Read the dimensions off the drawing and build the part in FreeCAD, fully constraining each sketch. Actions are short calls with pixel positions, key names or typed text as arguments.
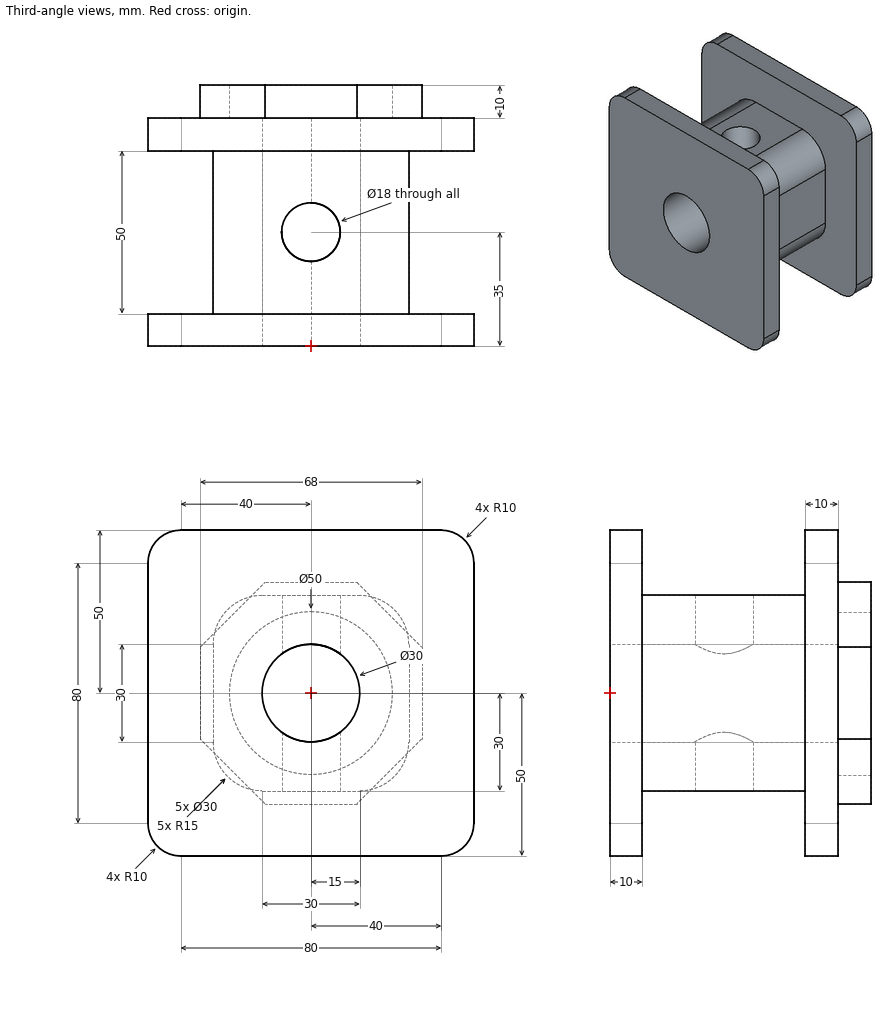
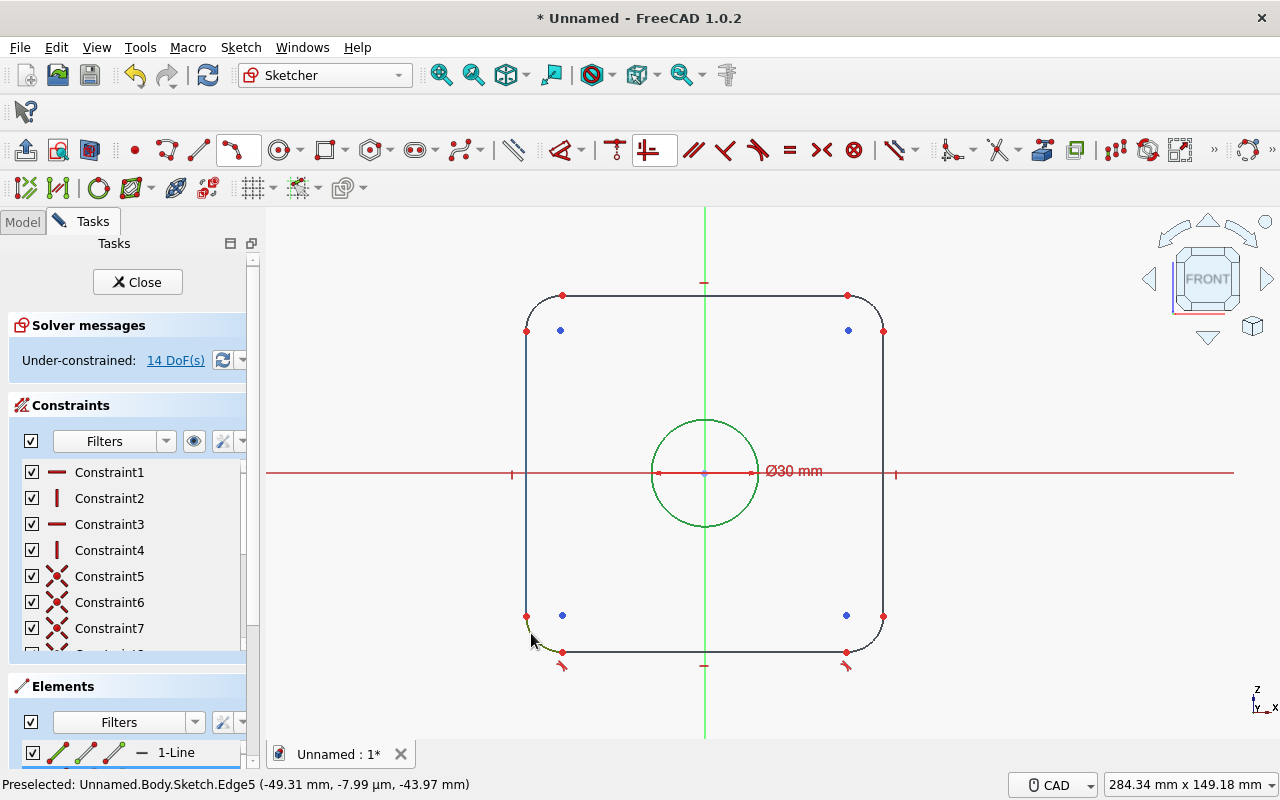
click(758, 150)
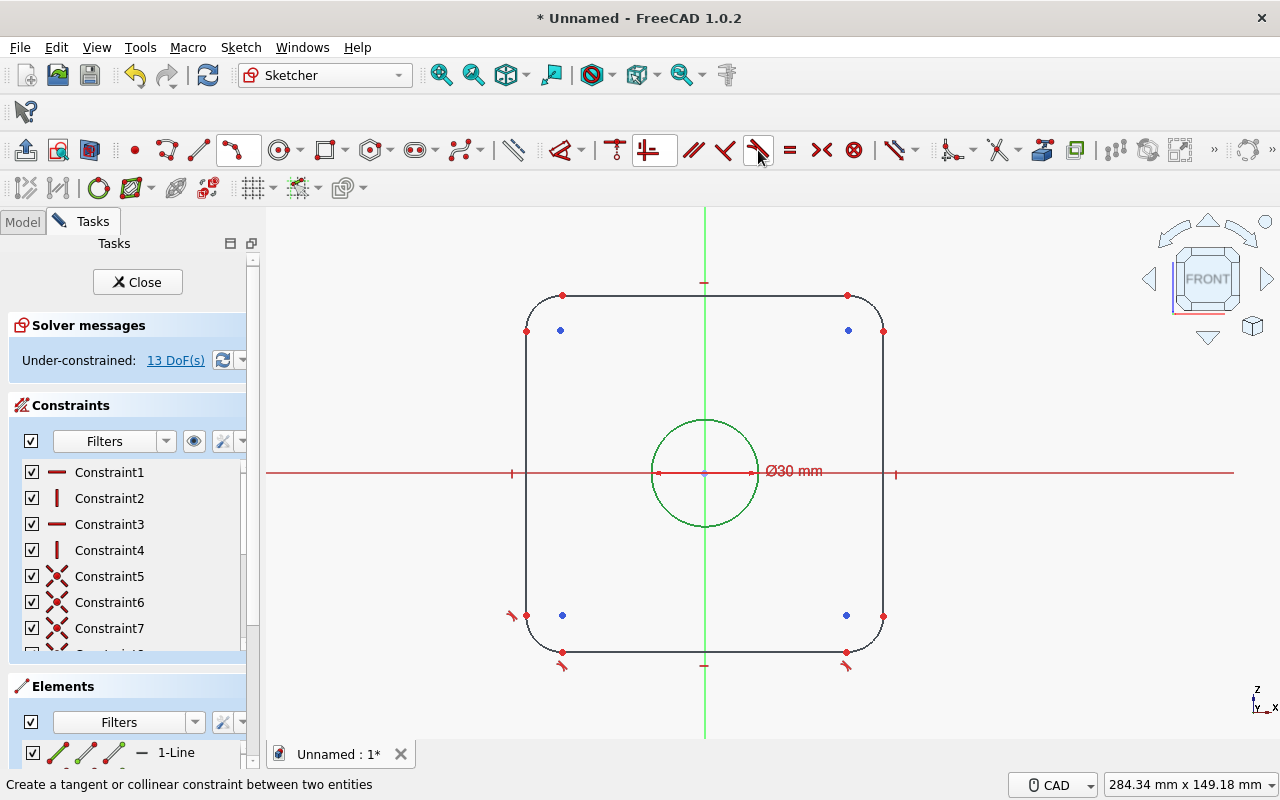
click(526, 531)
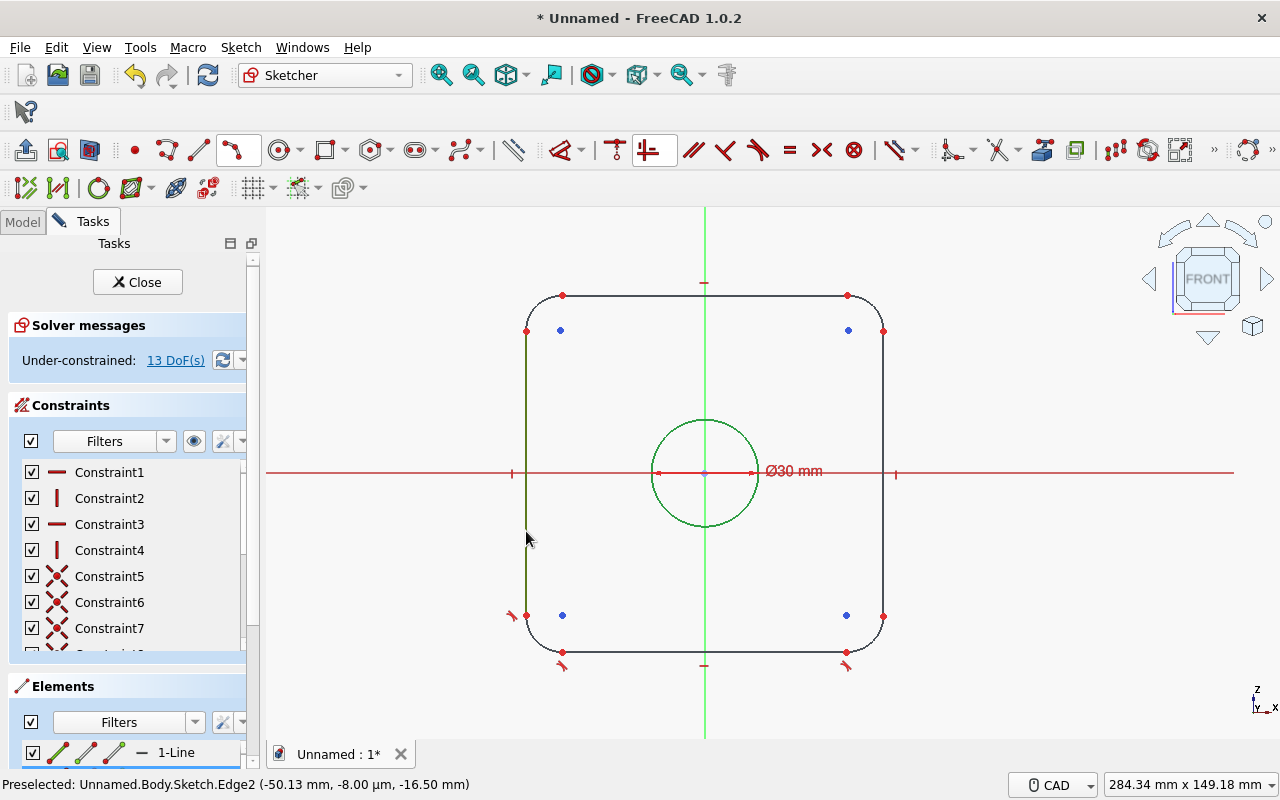
click(546, 299)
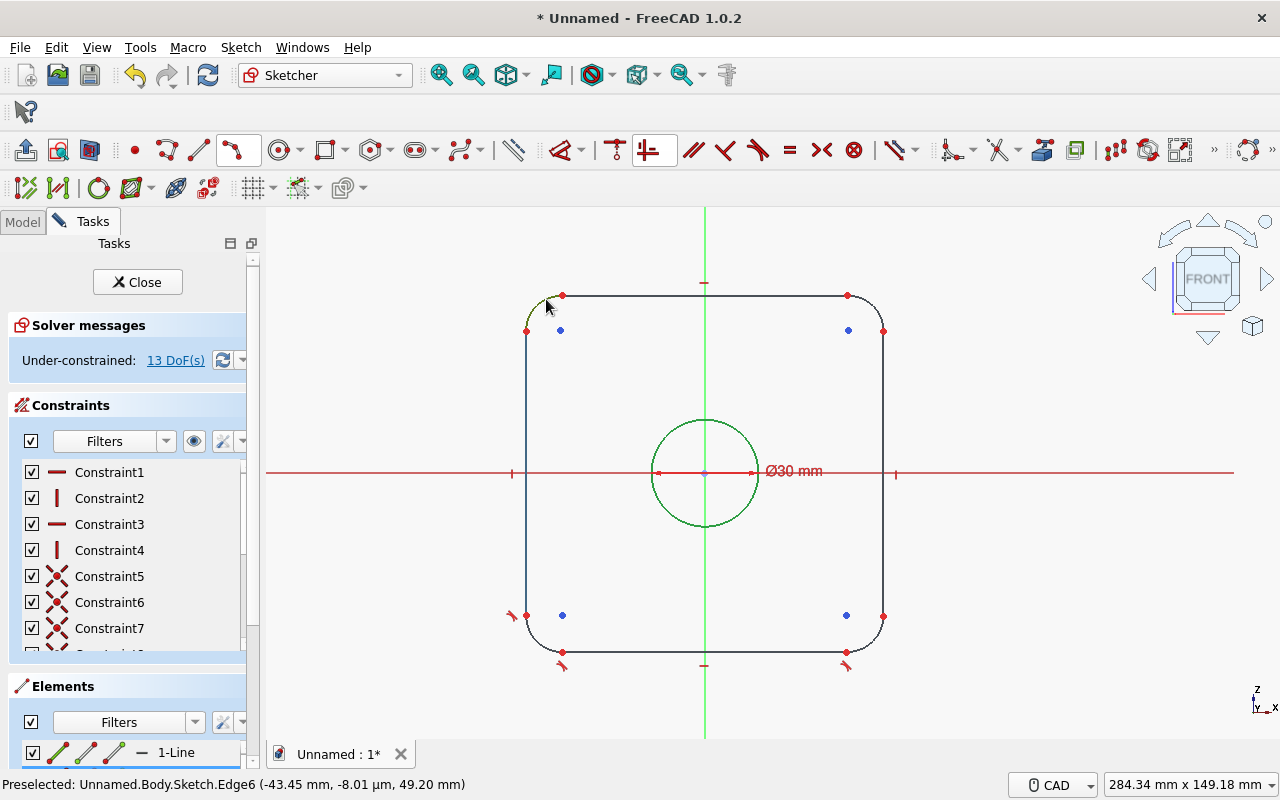
click(758, 150)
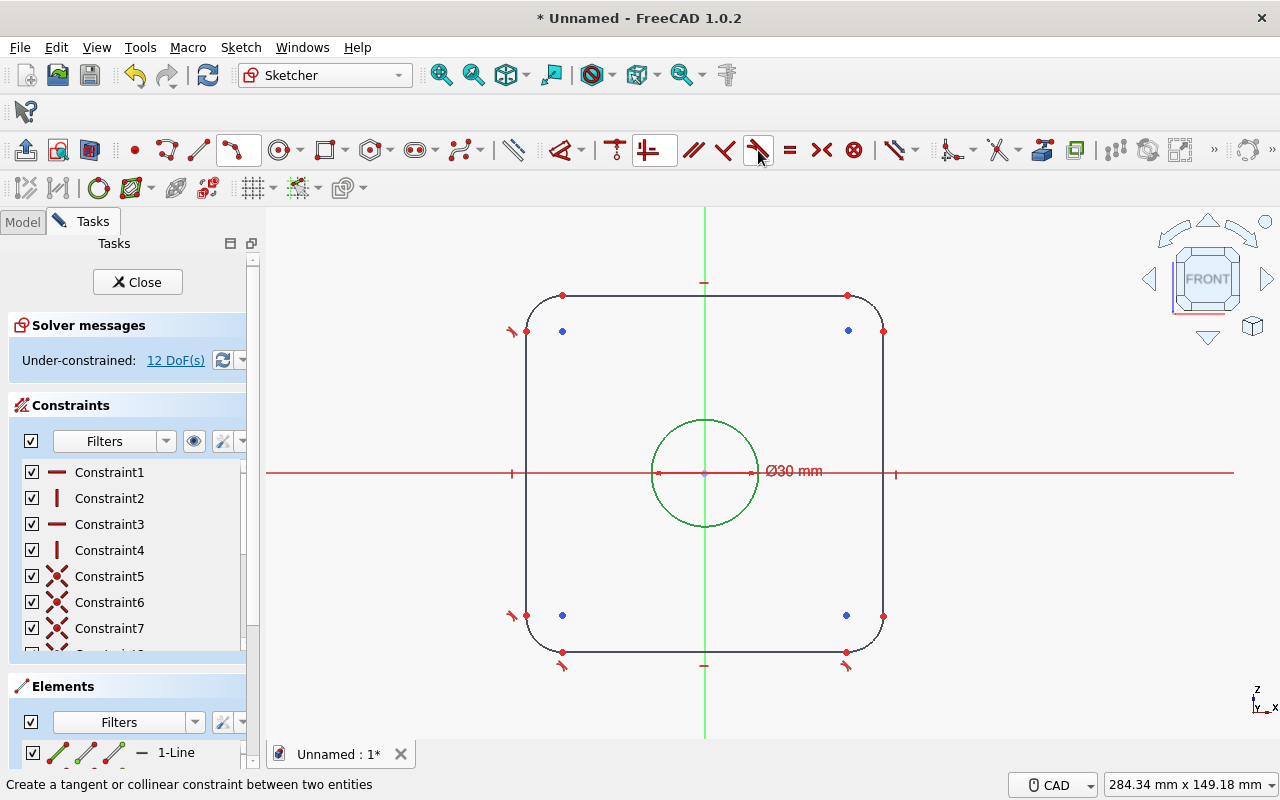
click(648, 296)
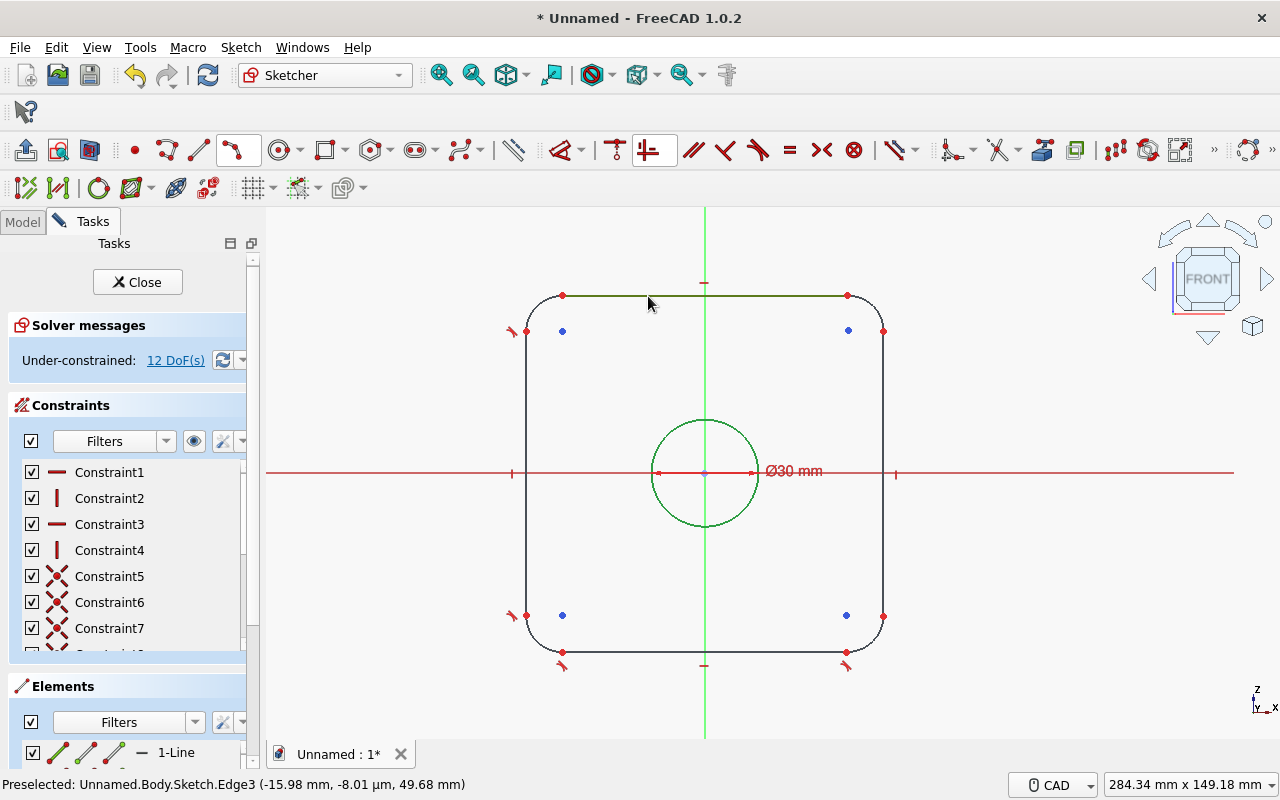
click(546, 300)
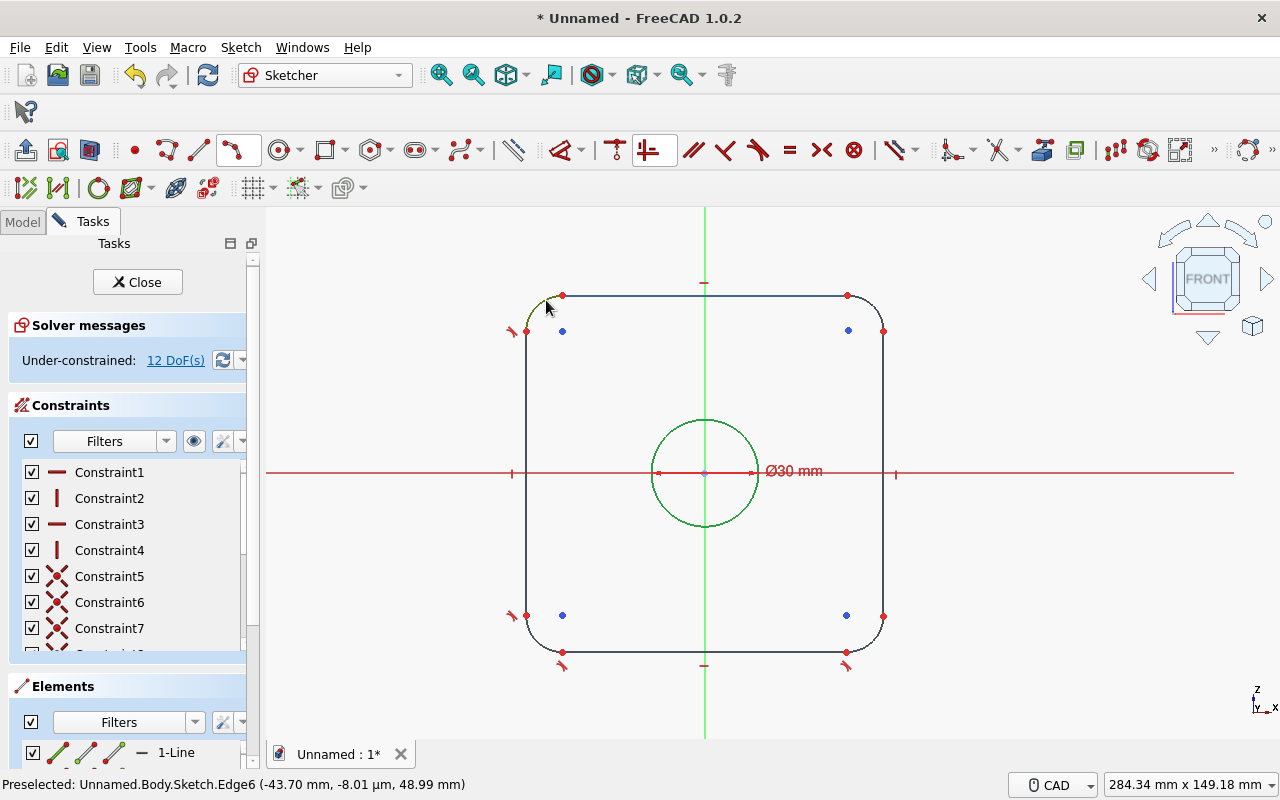
click(758, 150)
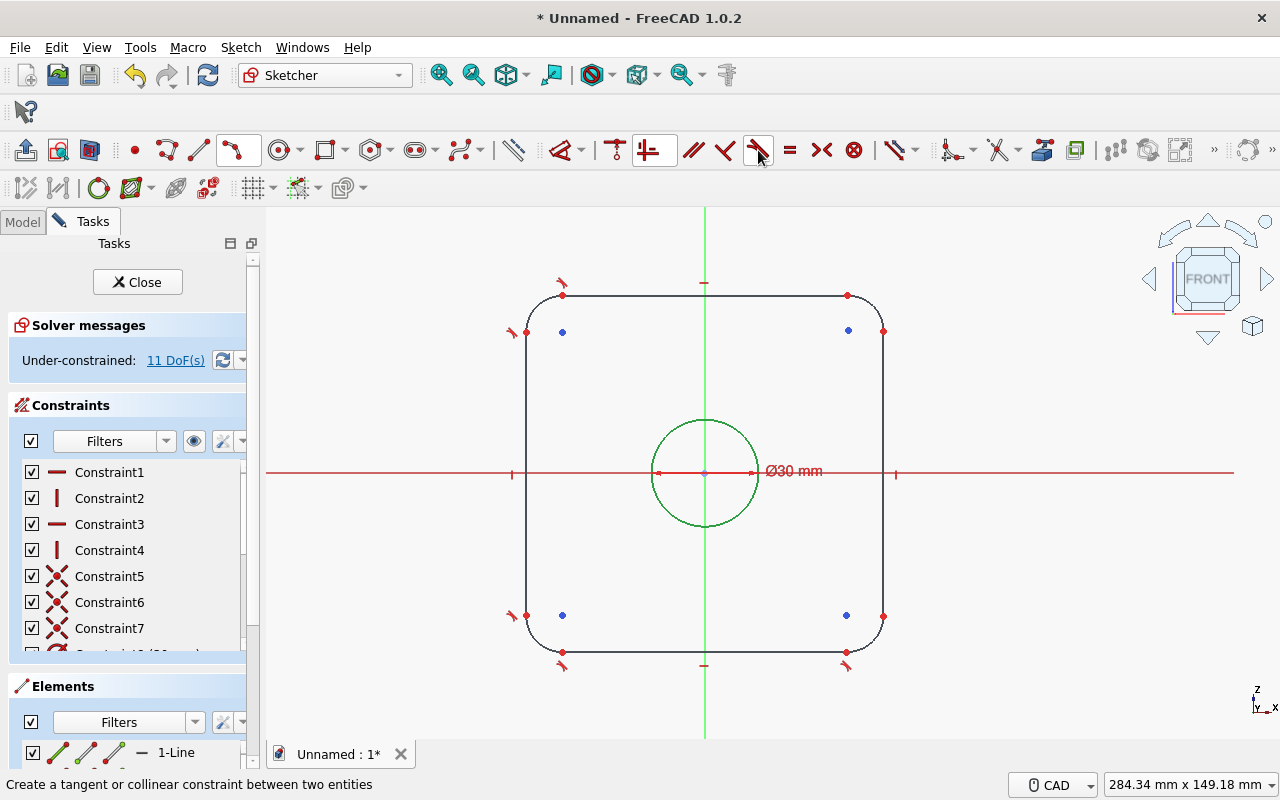
click(648, 296)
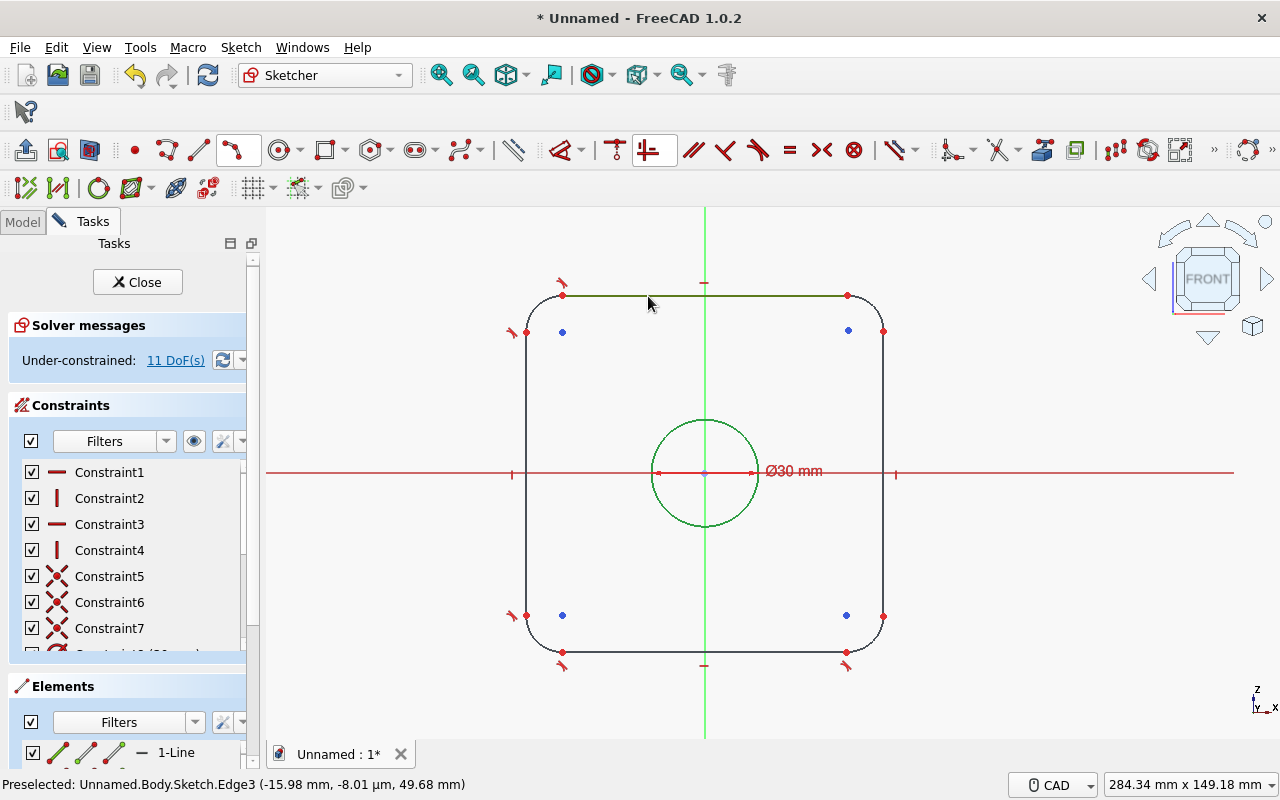
click(880, 315)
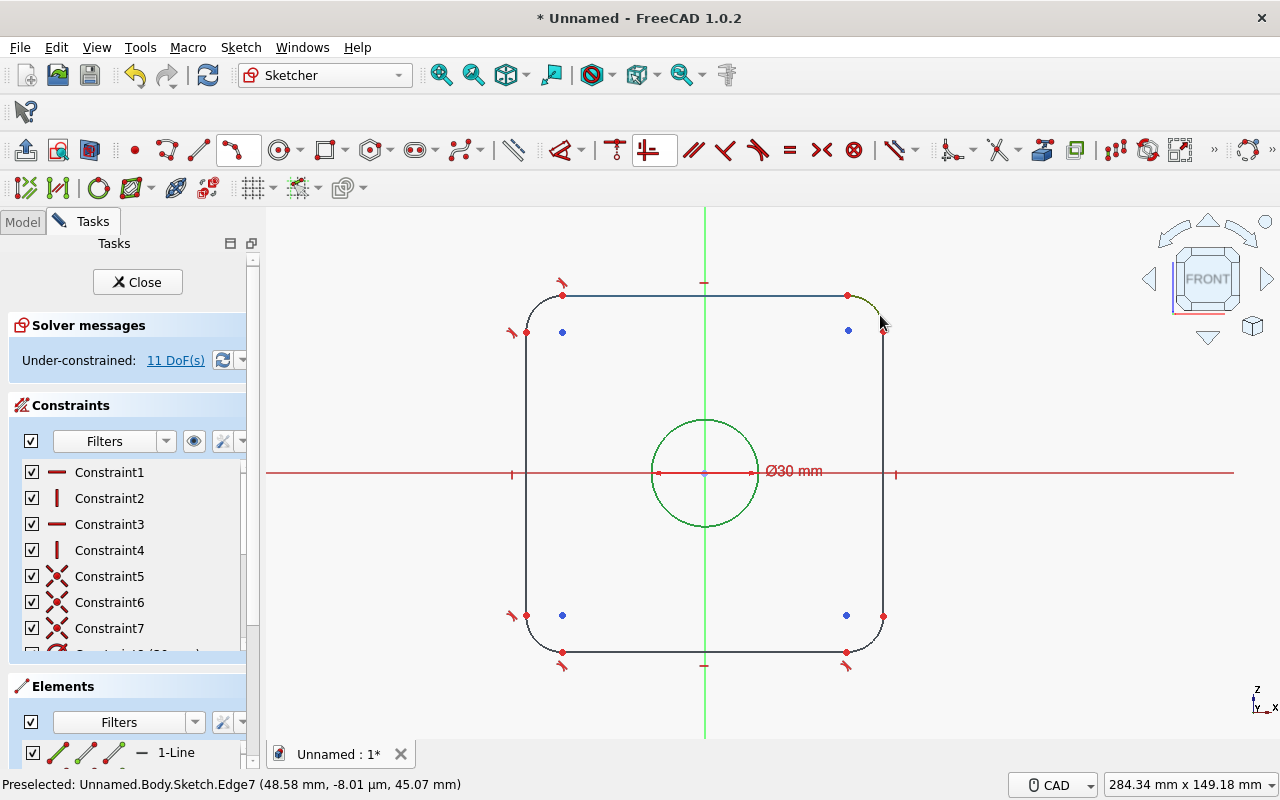
click(758, 150)